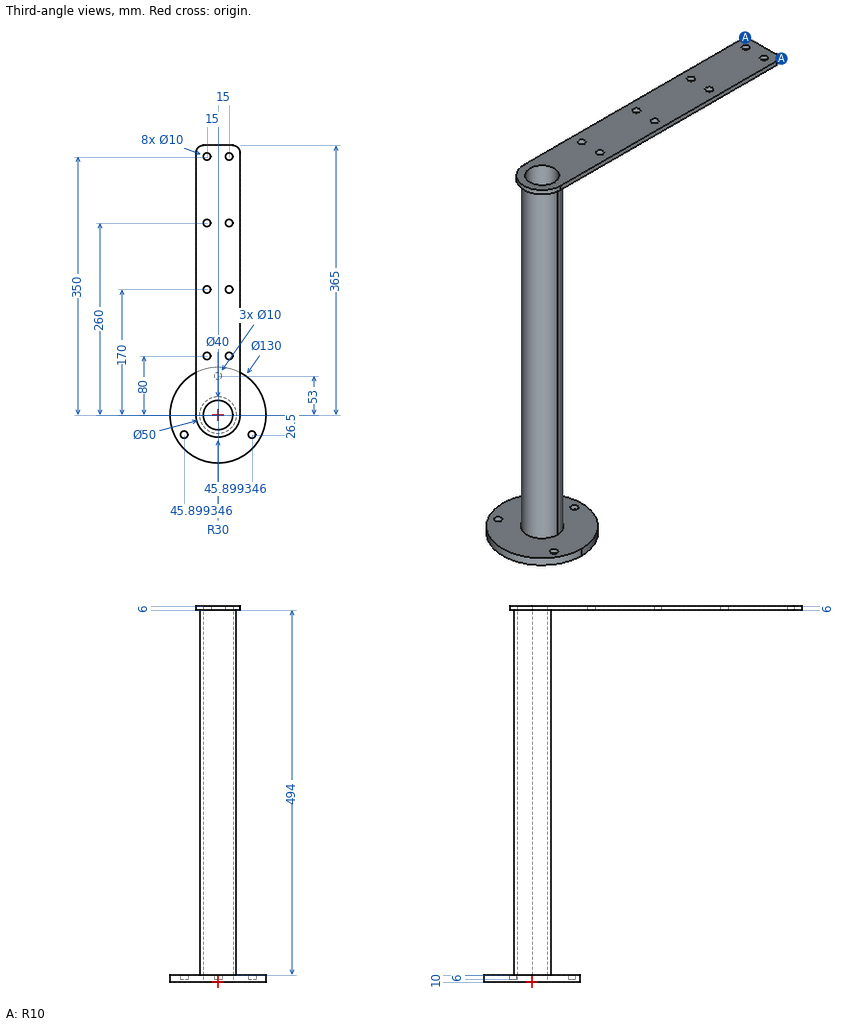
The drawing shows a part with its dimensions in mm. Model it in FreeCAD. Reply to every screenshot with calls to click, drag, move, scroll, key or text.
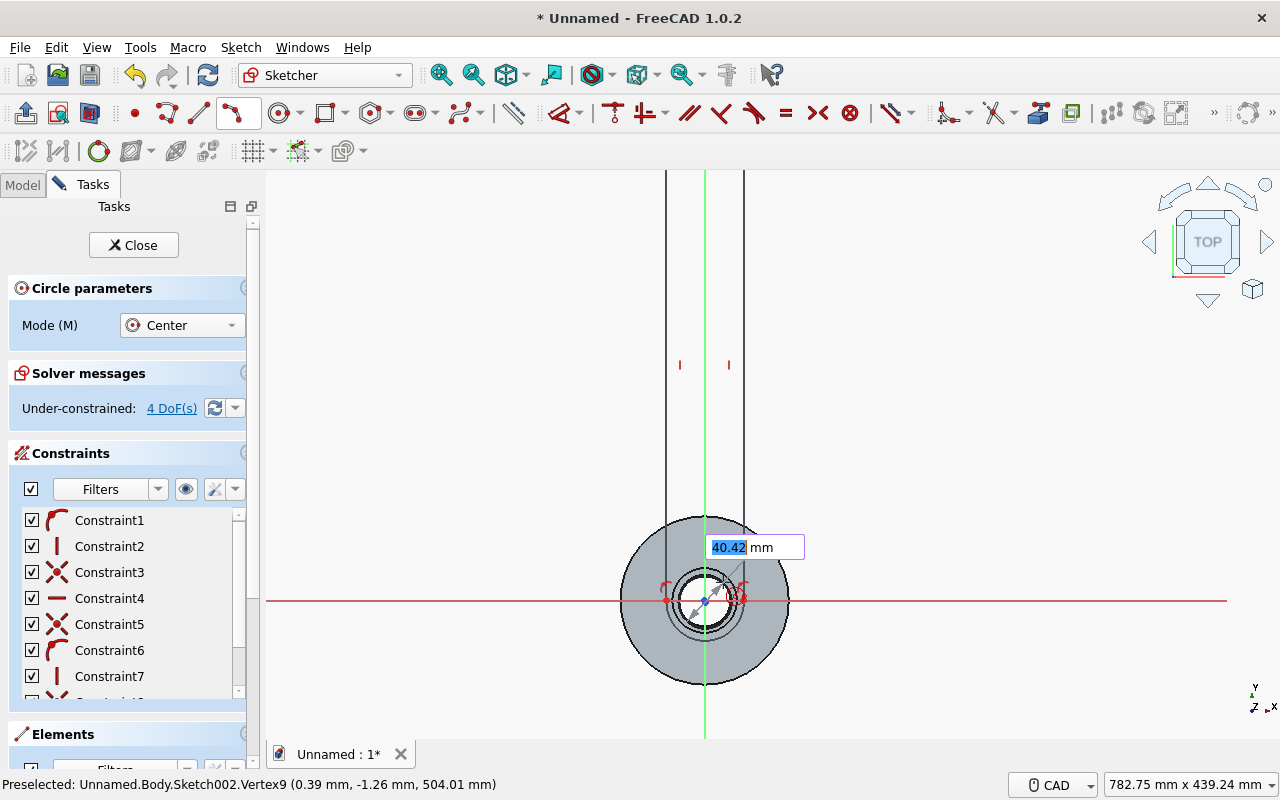
text(40)
key(Return)
key(Escape)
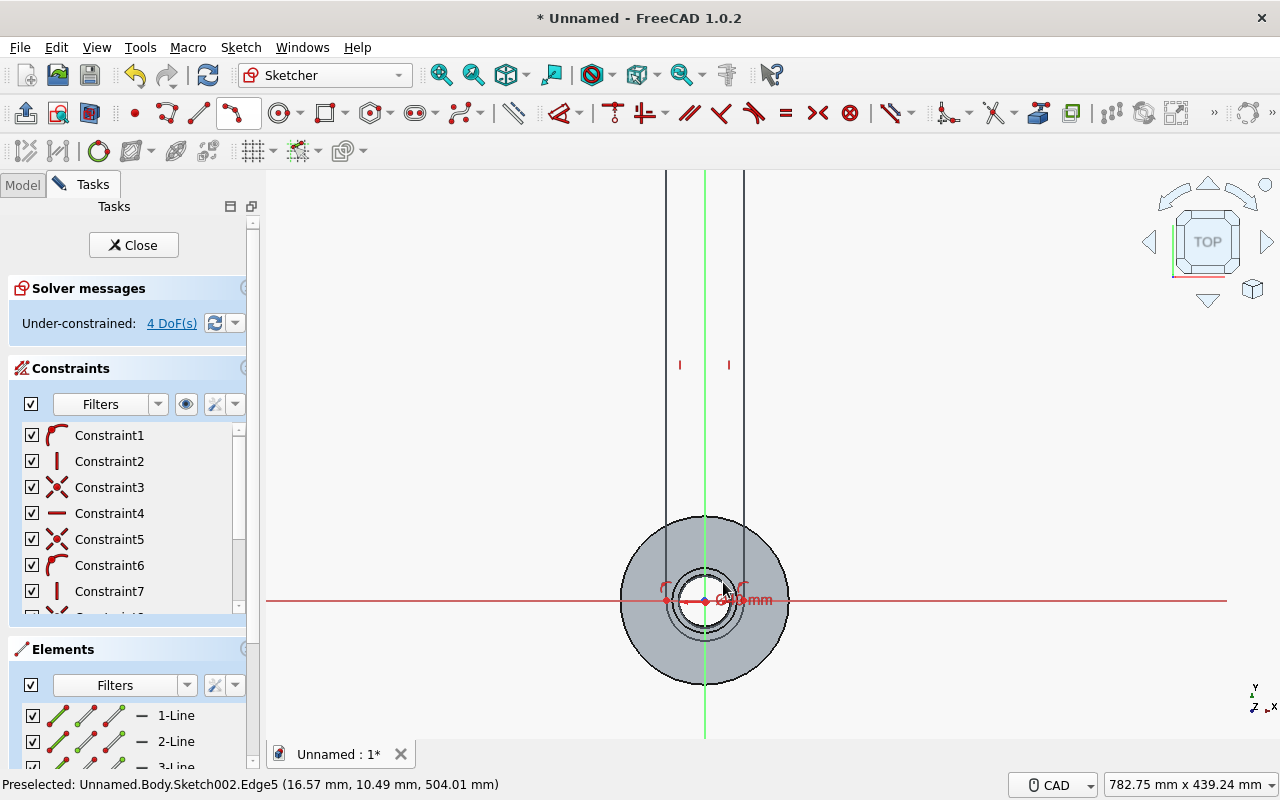
scroll(705, 601, up, 3)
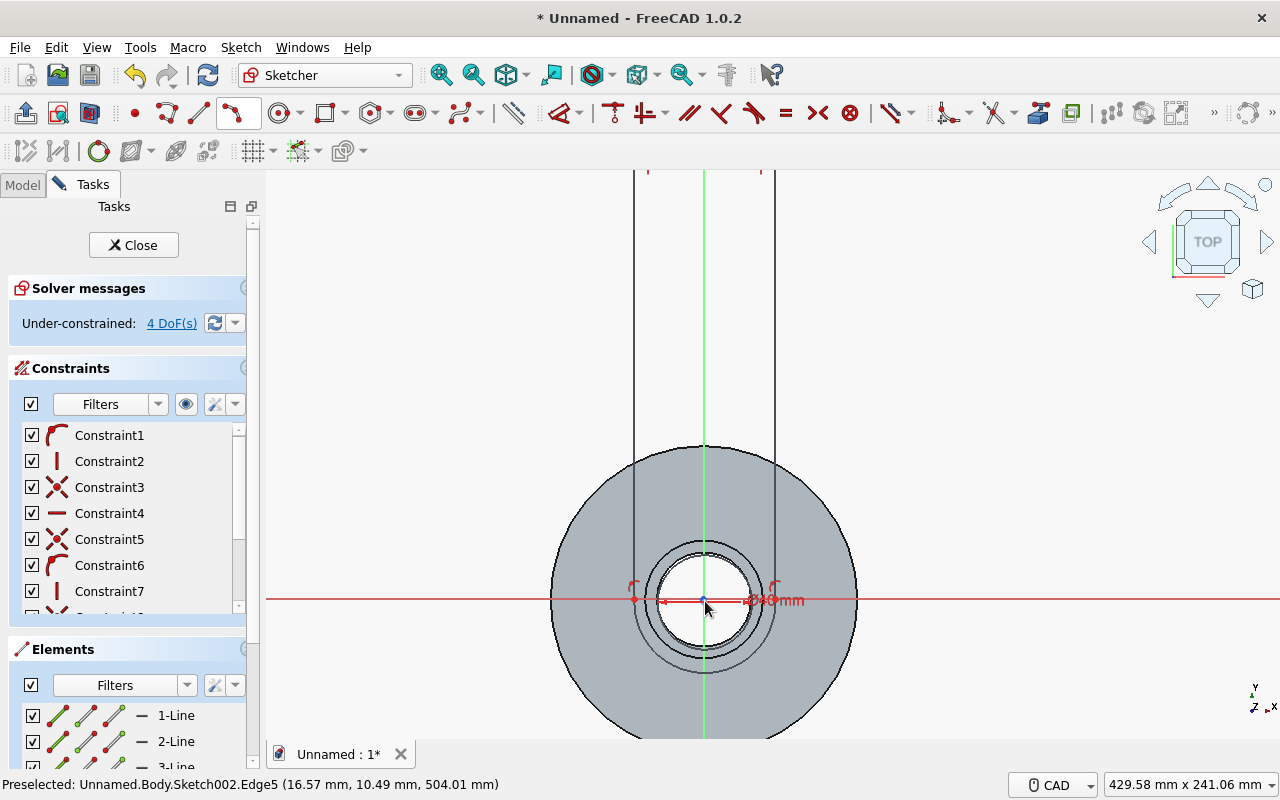
drag(694, 589, 715, 612)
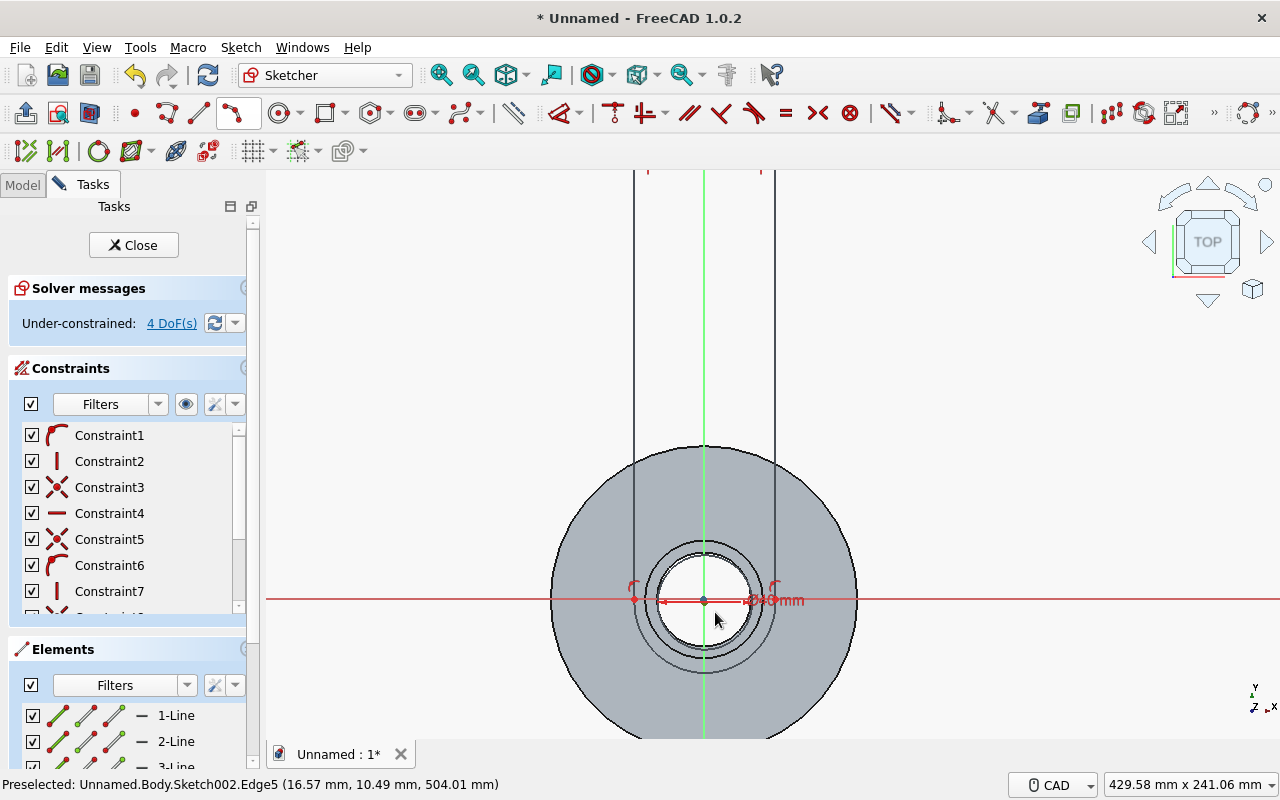
click(614, 114)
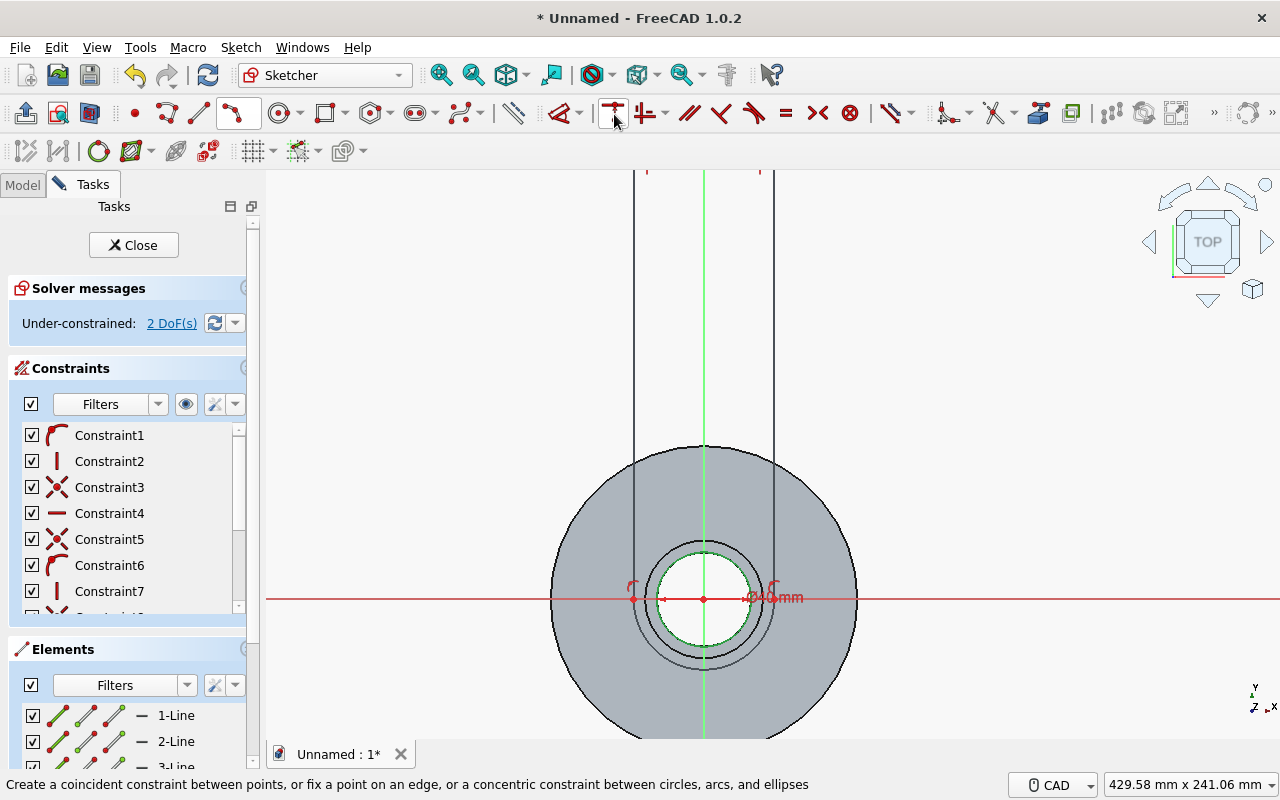
click(560, 114)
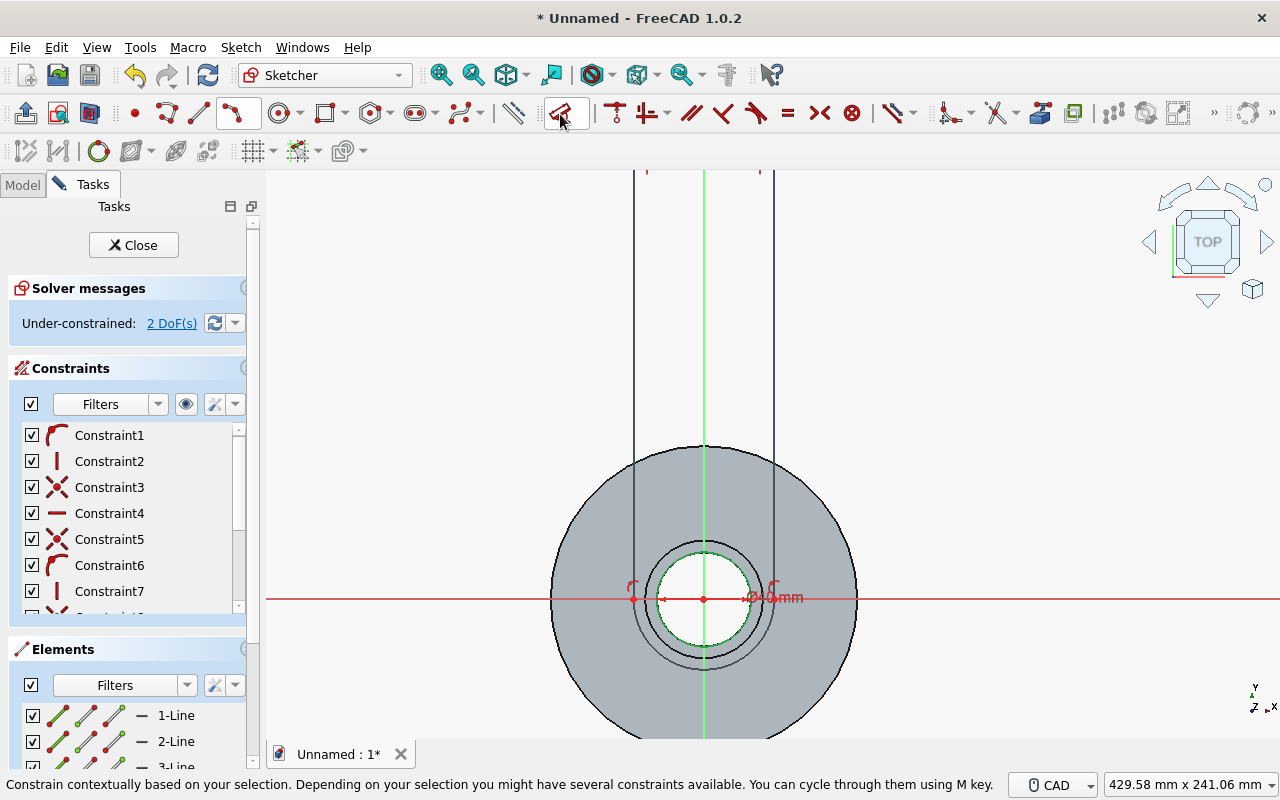
click(663, 656)
click(644, 682)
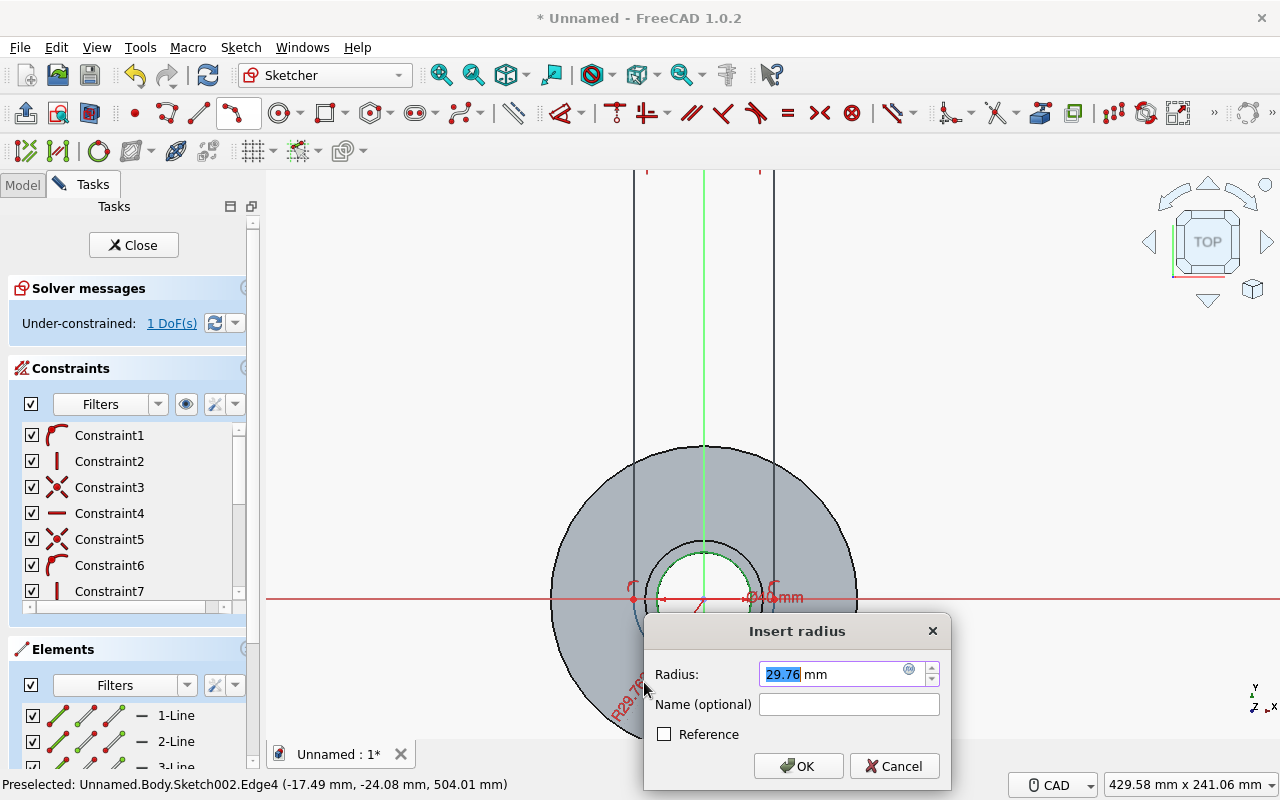
text(30)
key(Return)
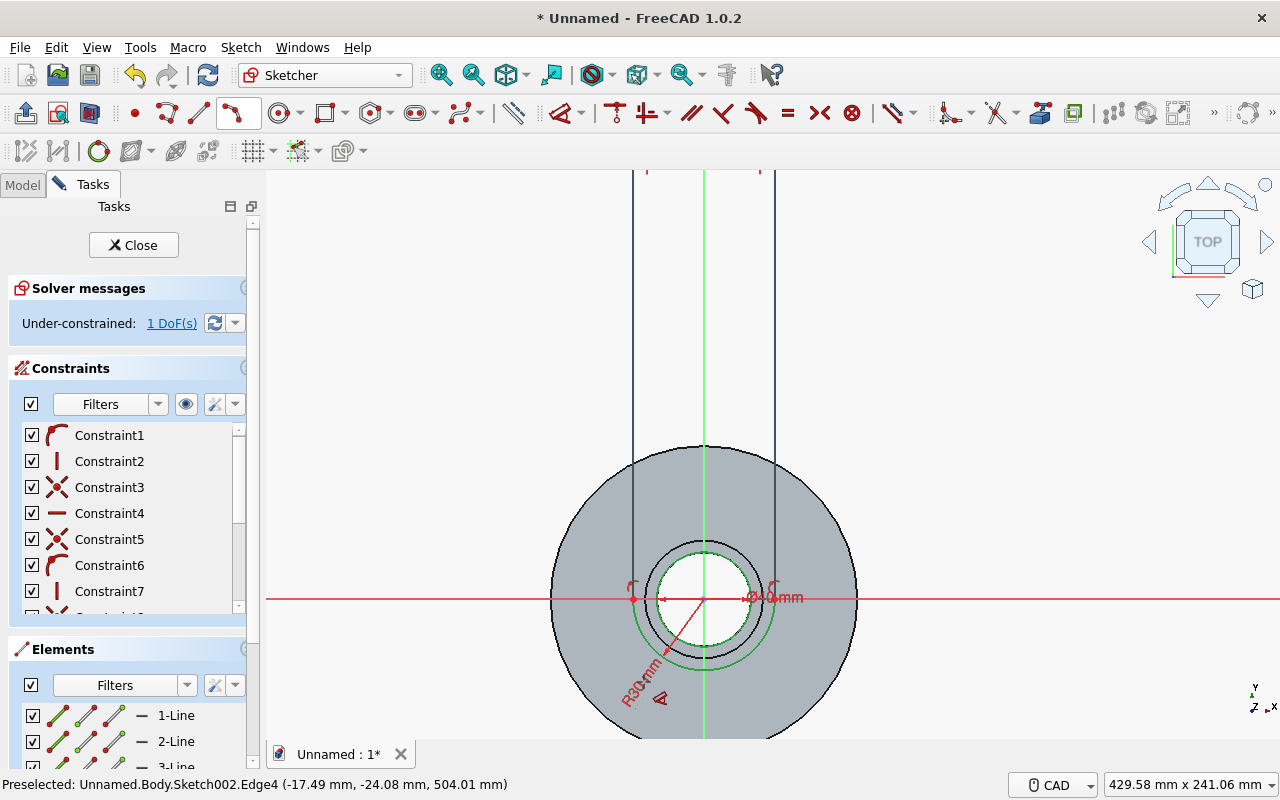
click(775, 342)
click(809, 399)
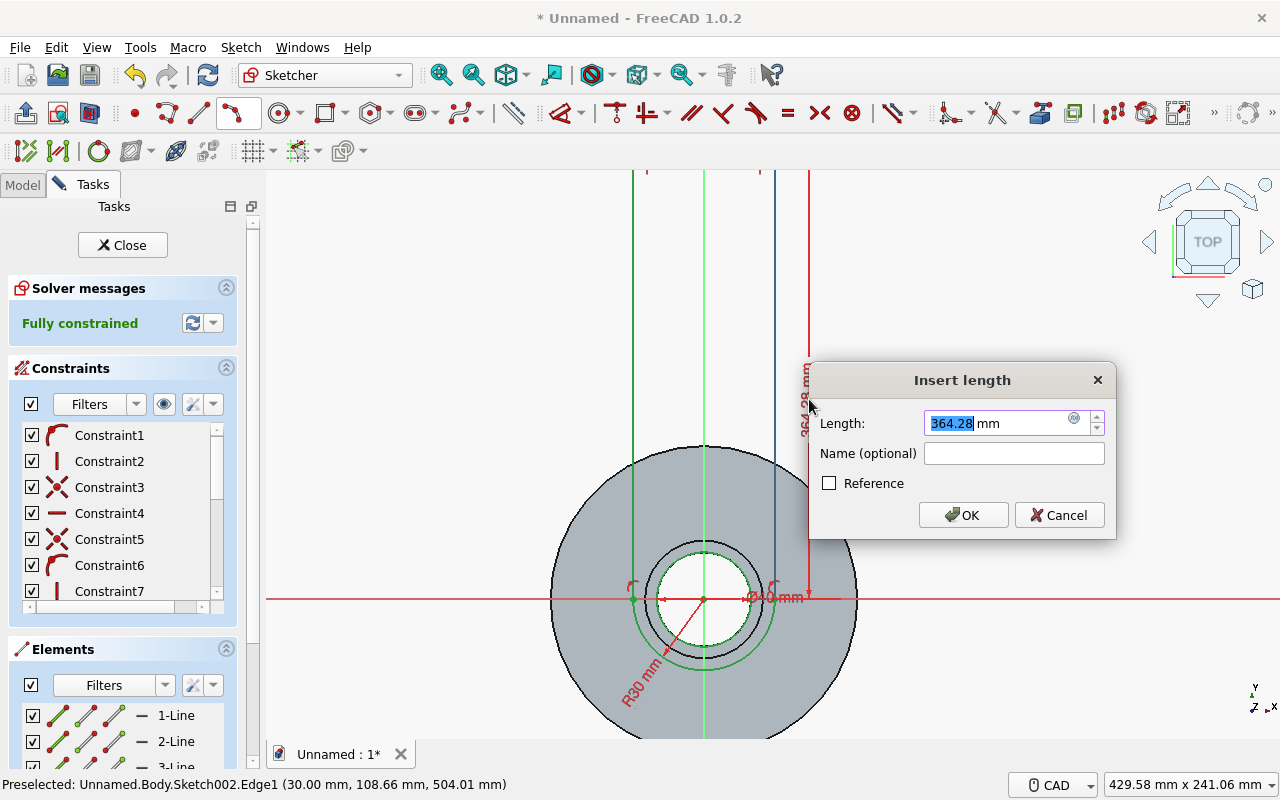
text(365)
key(Return)
key(Escape)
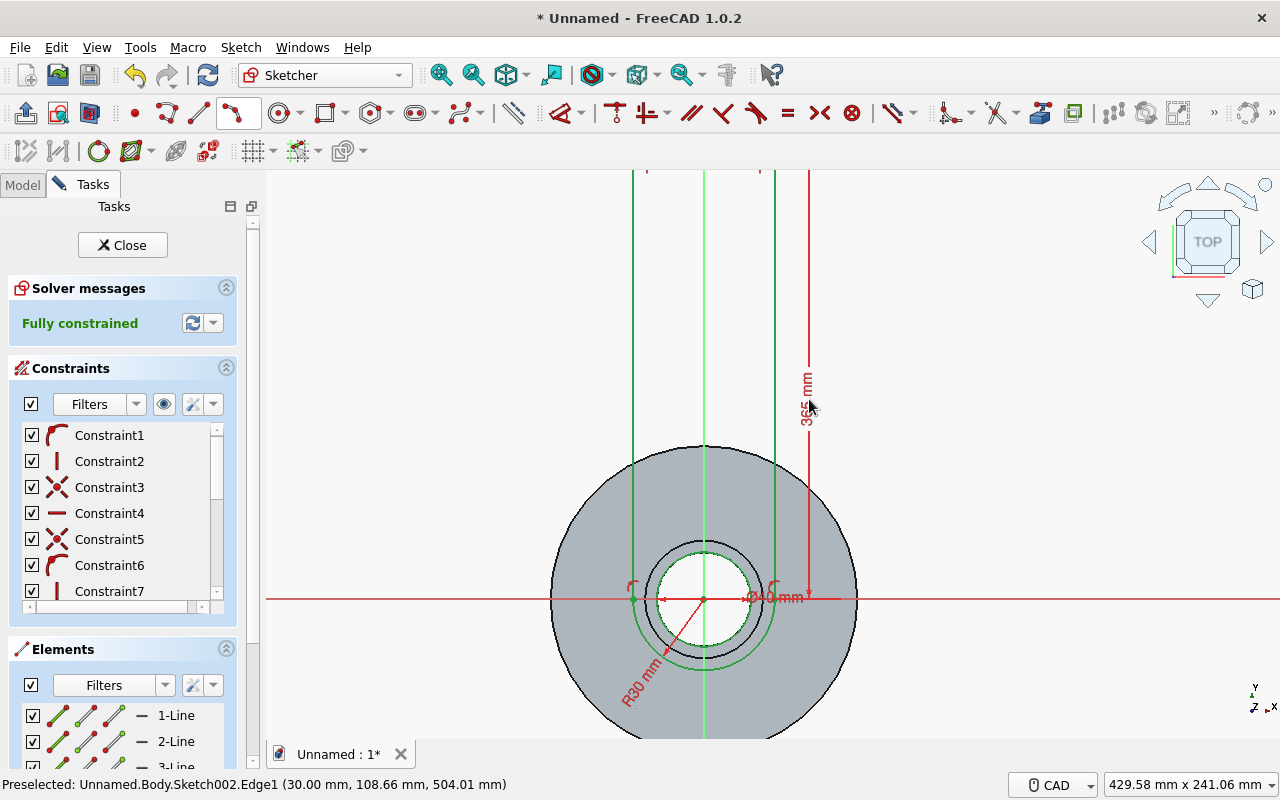
click(123, 245)